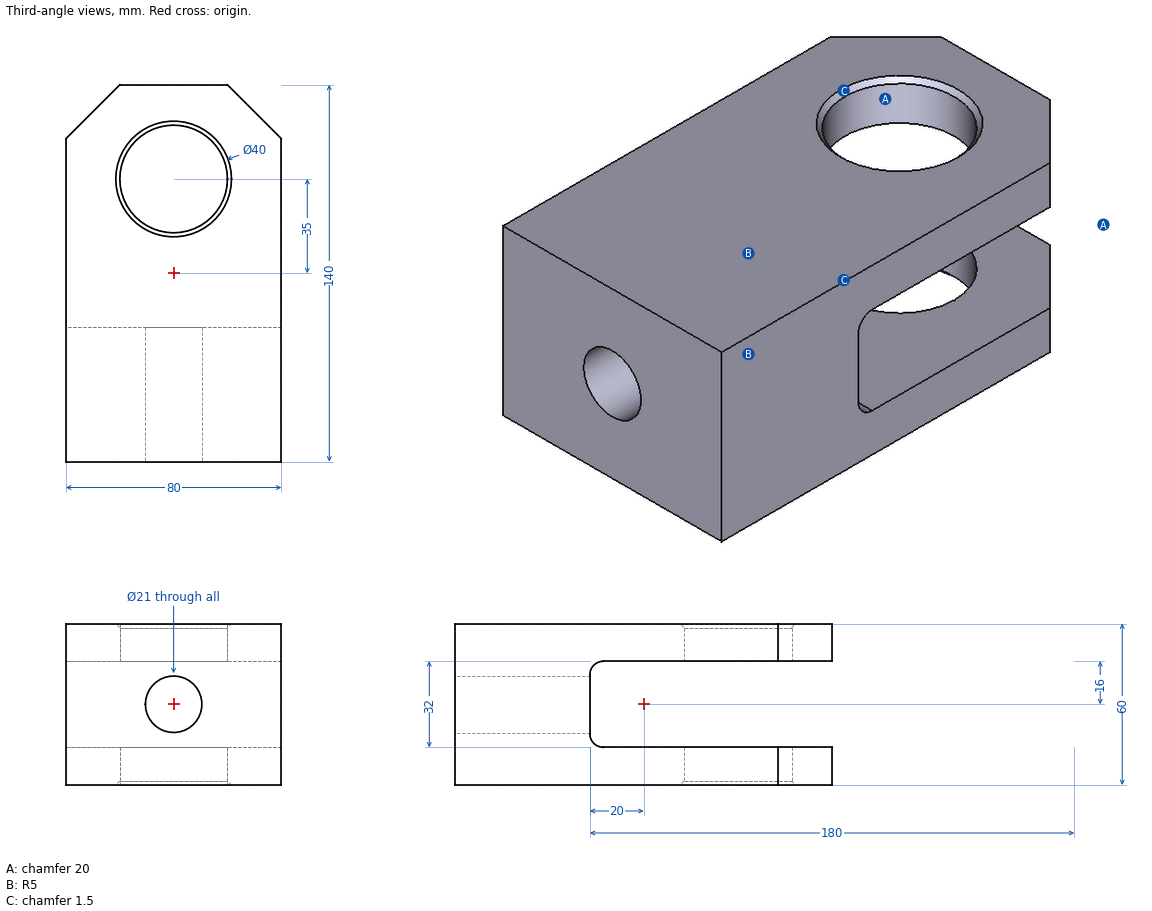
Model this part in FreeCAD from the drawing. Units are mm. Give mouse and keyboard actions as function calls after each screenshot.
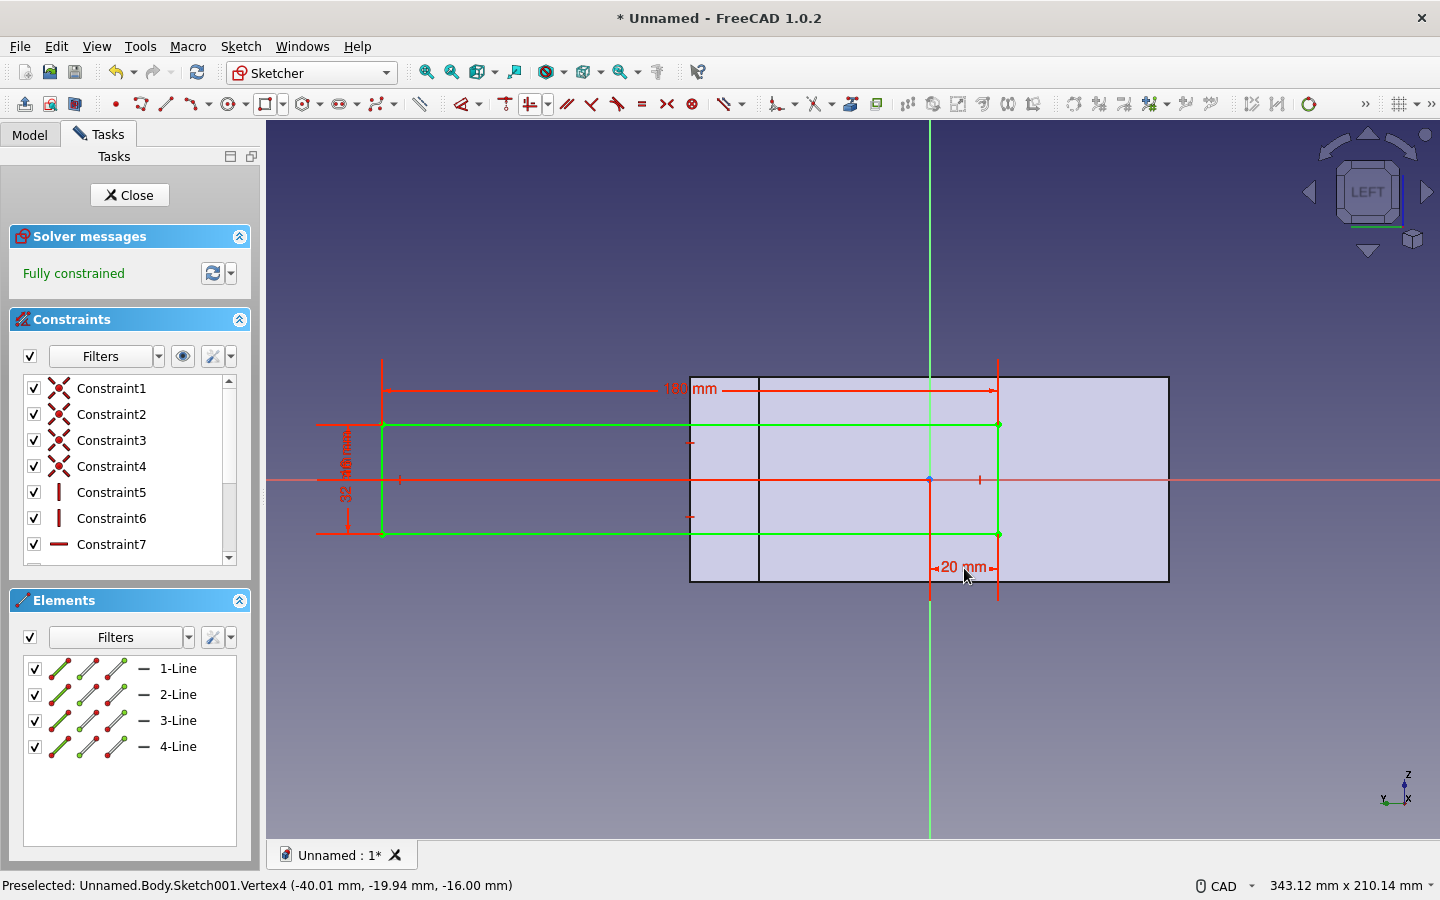
click(130, 195)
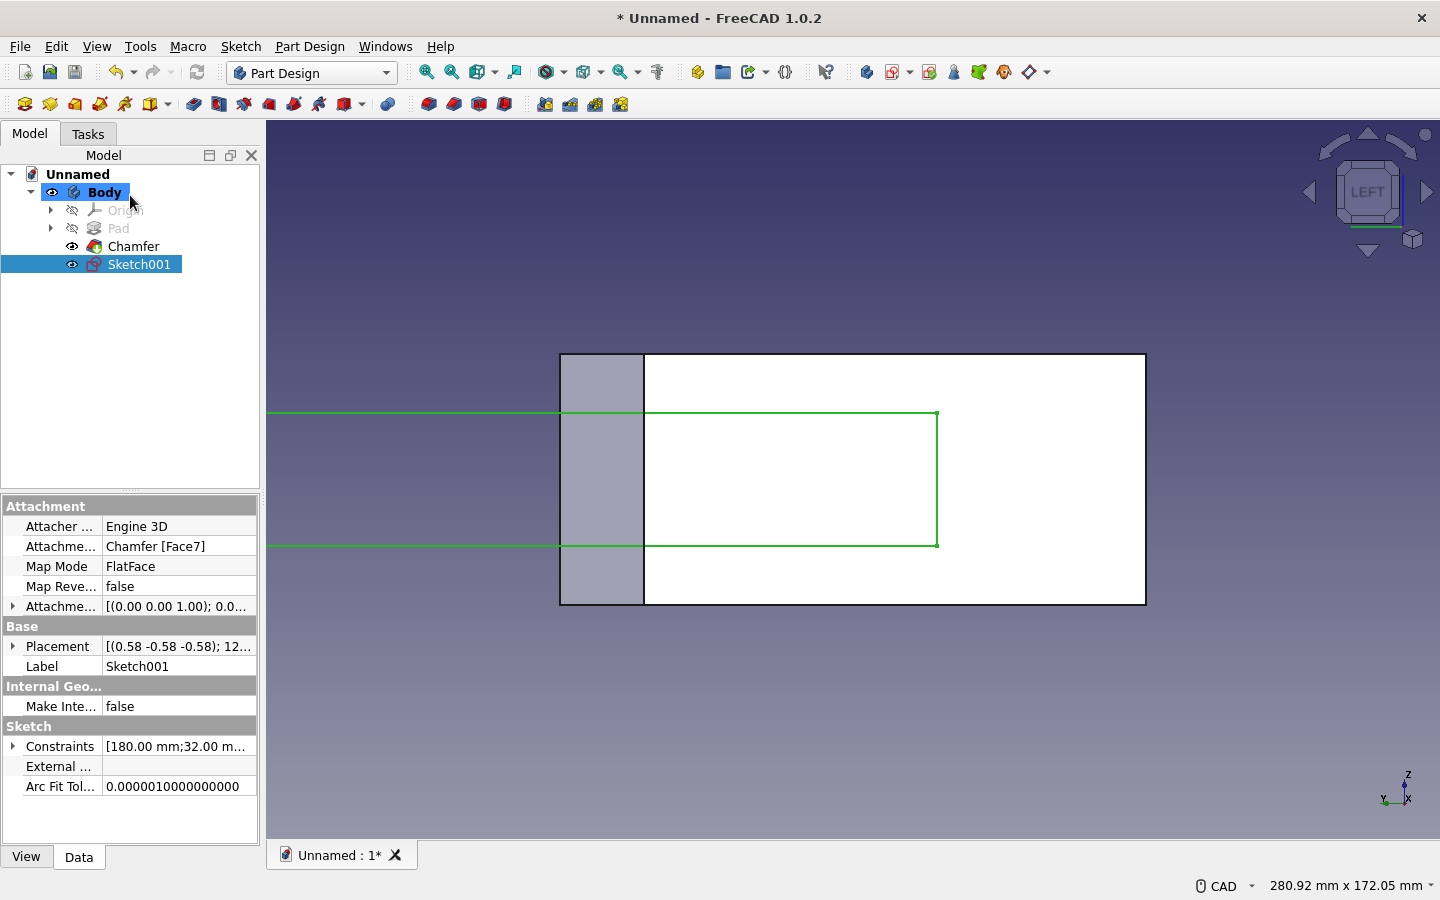
click(194, 104)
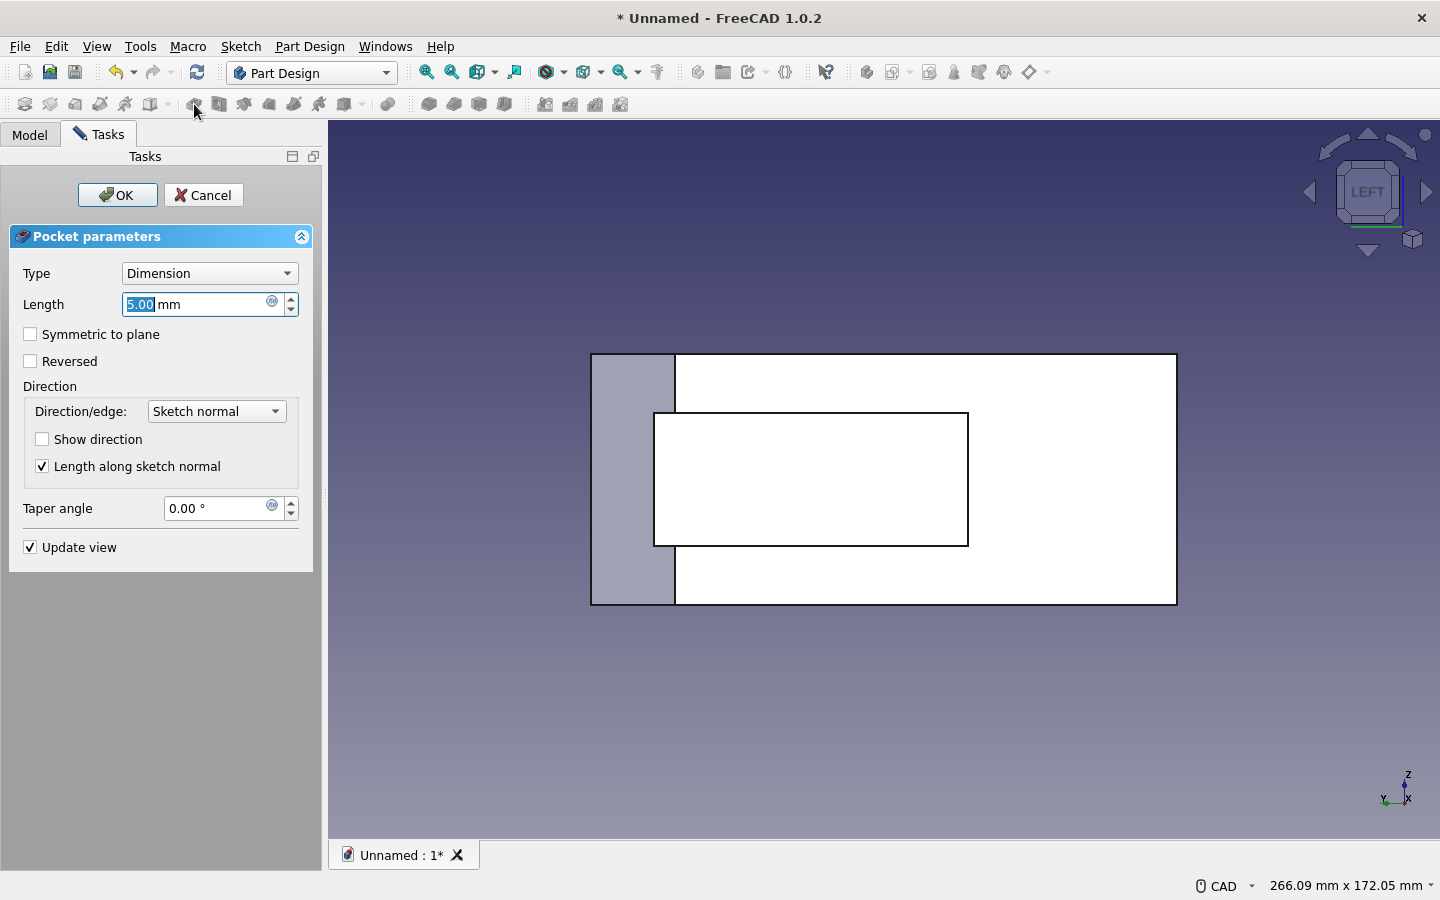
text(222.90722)
key(Tab)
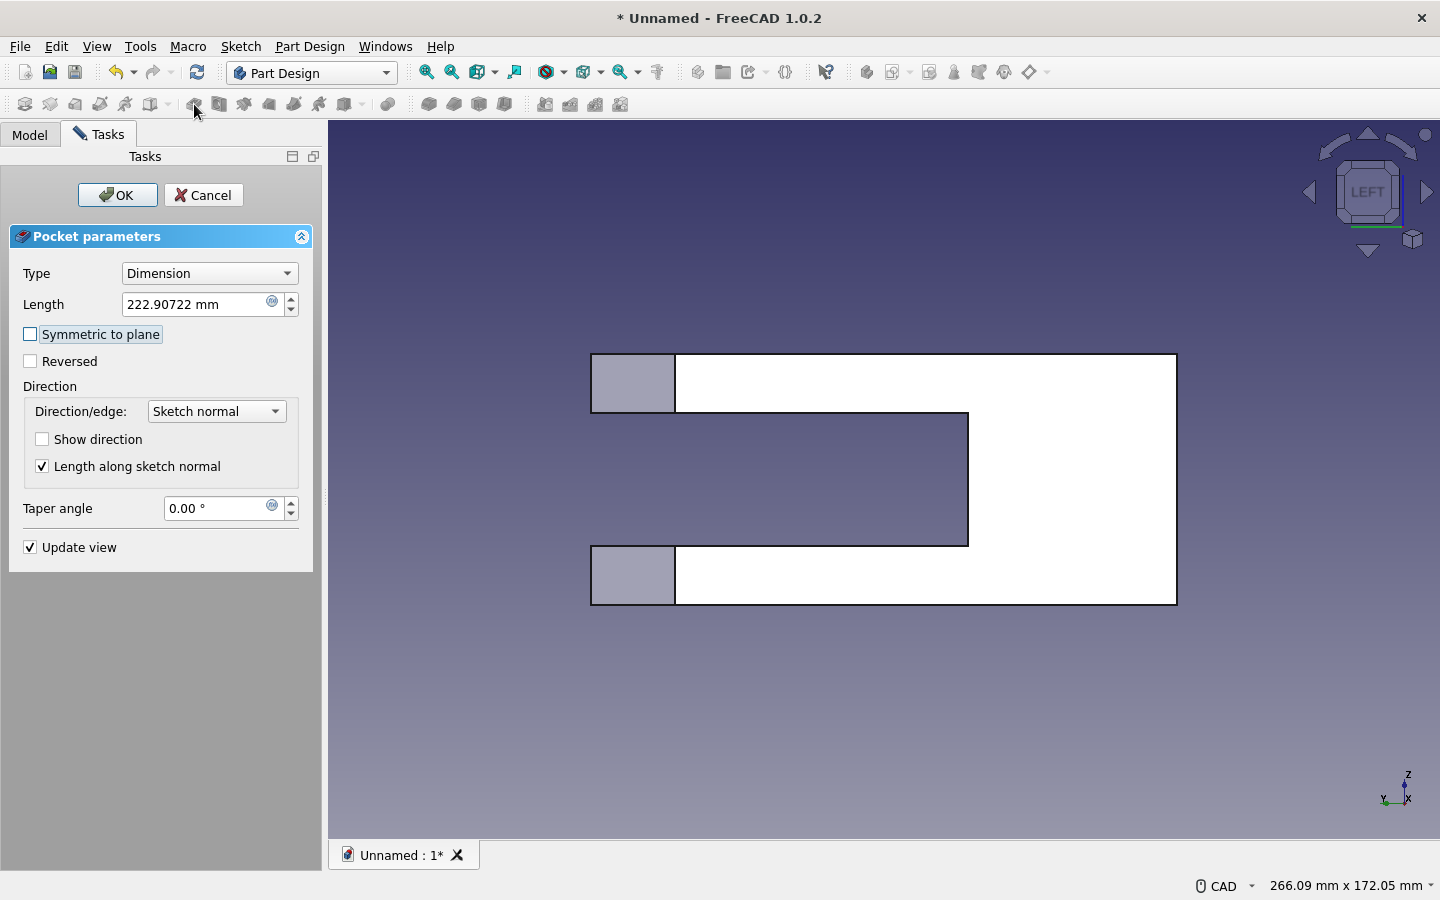
click(31, 334)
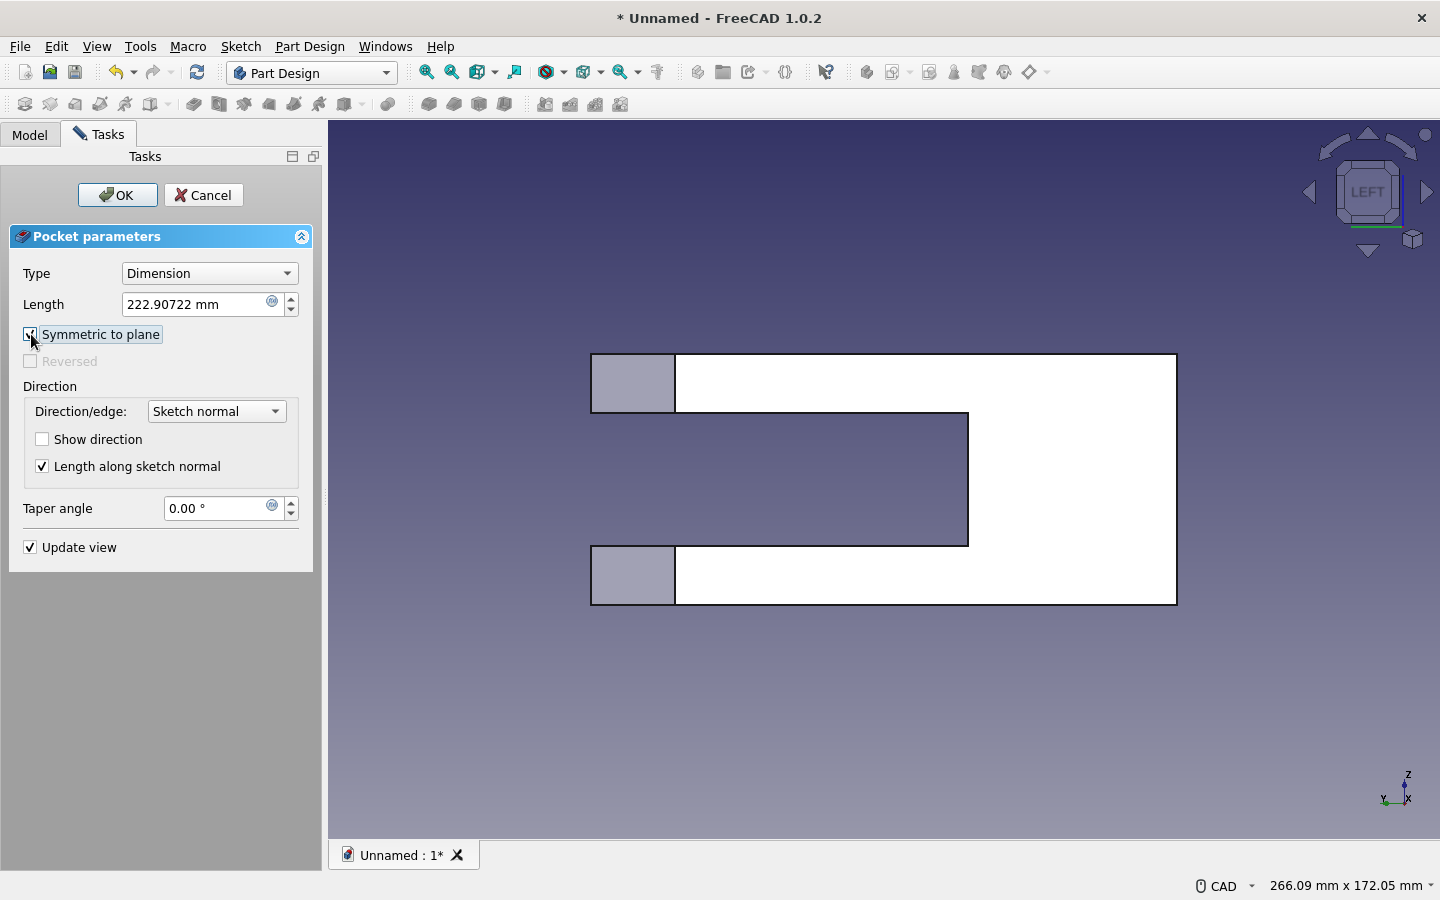
click(118, 195)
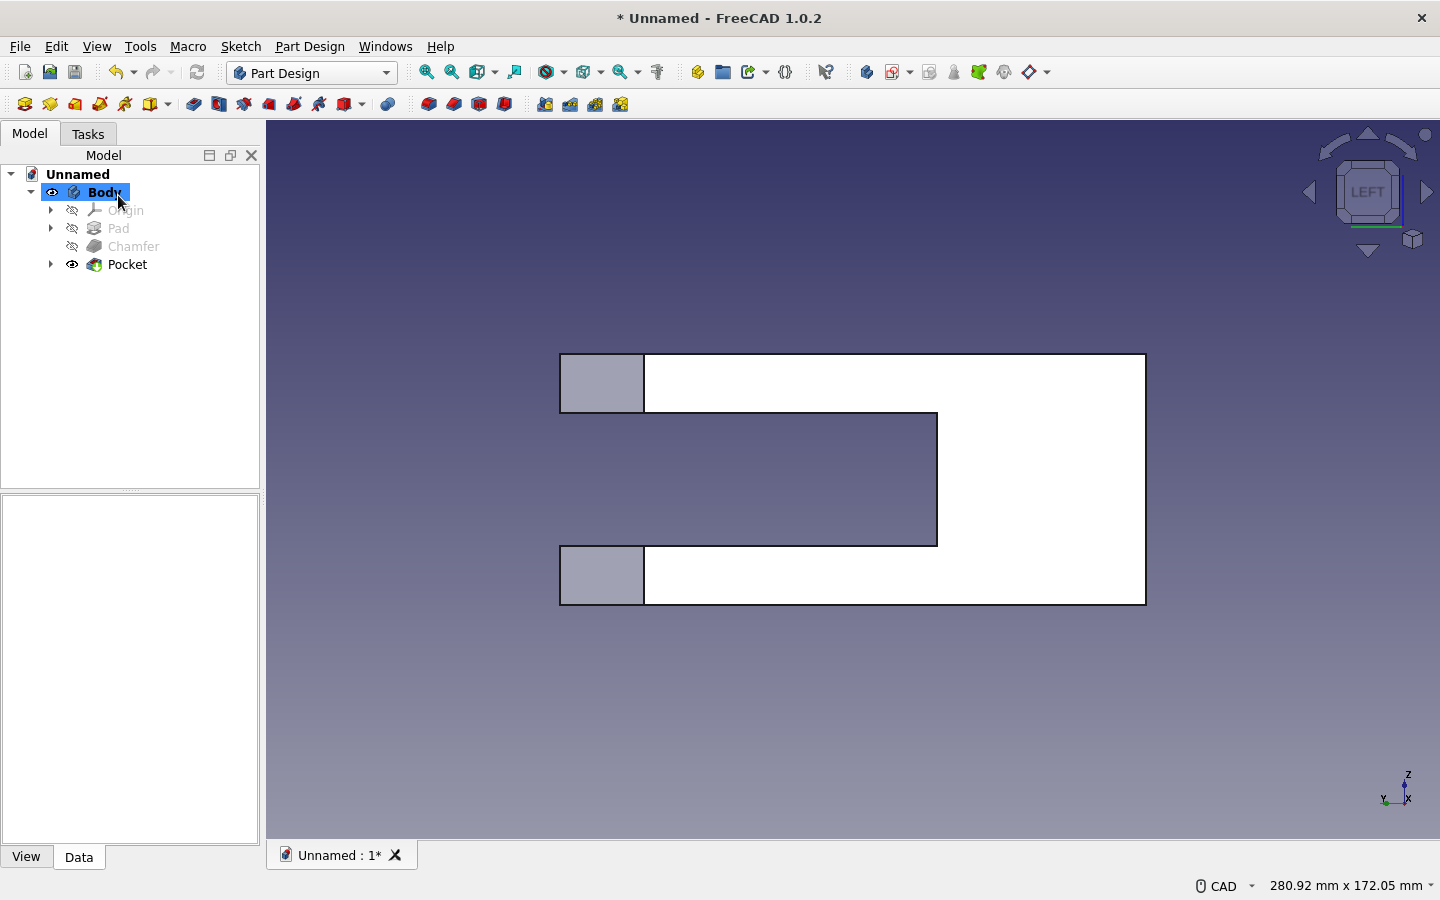
key(0)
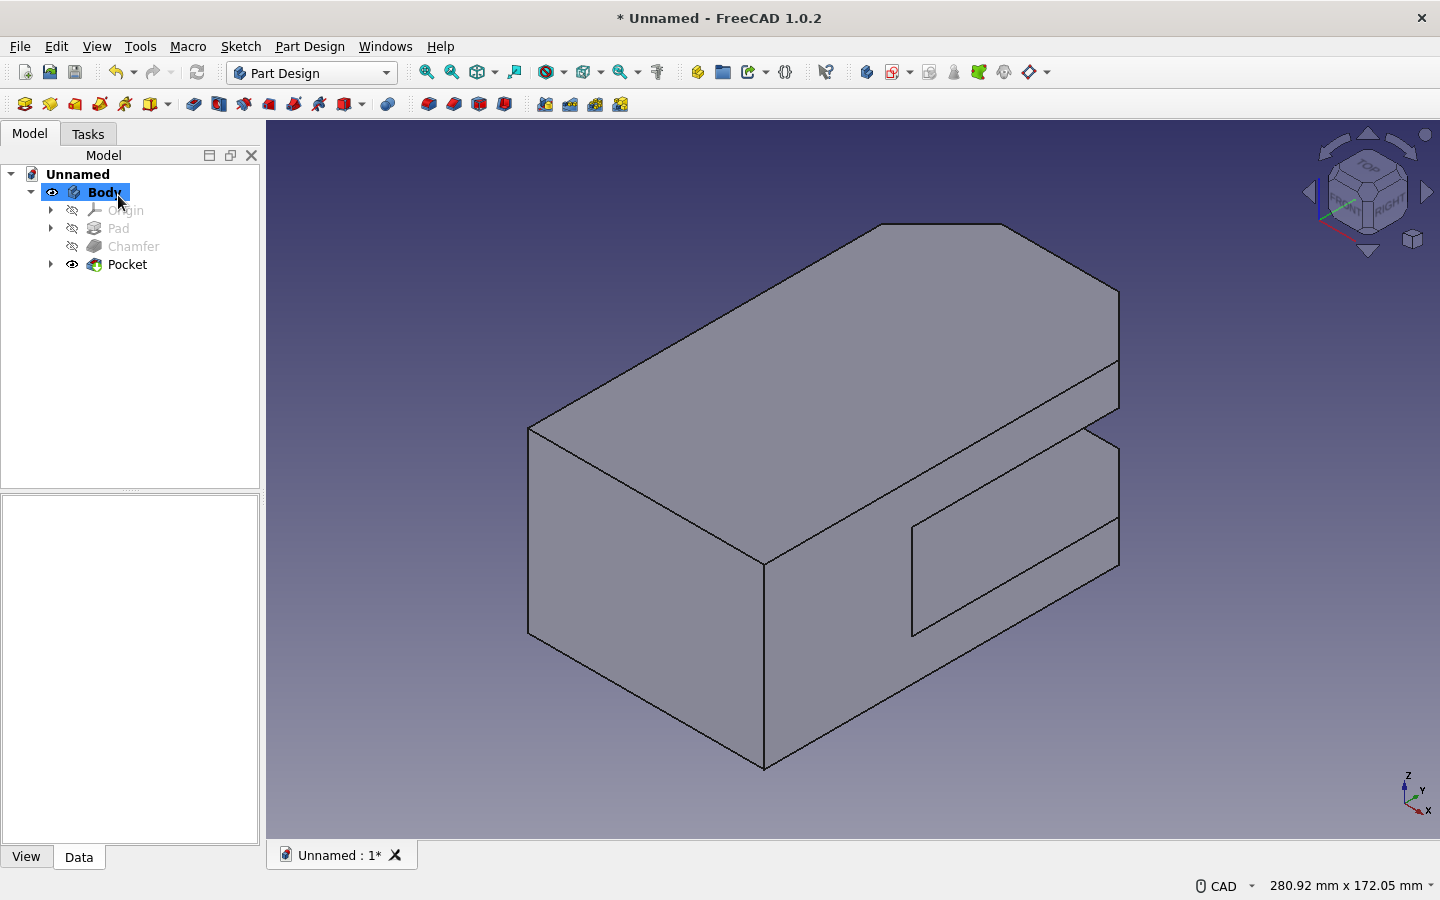
key(2)